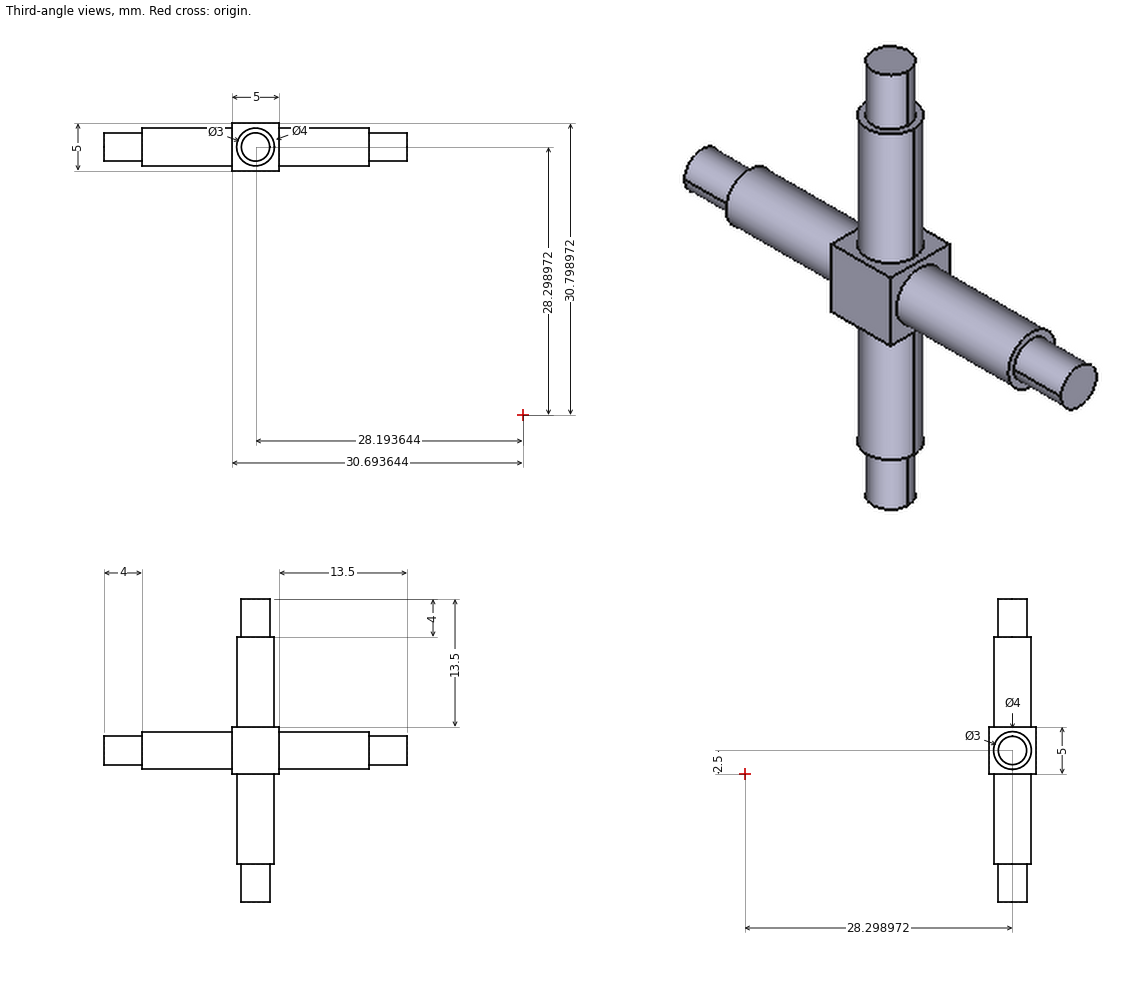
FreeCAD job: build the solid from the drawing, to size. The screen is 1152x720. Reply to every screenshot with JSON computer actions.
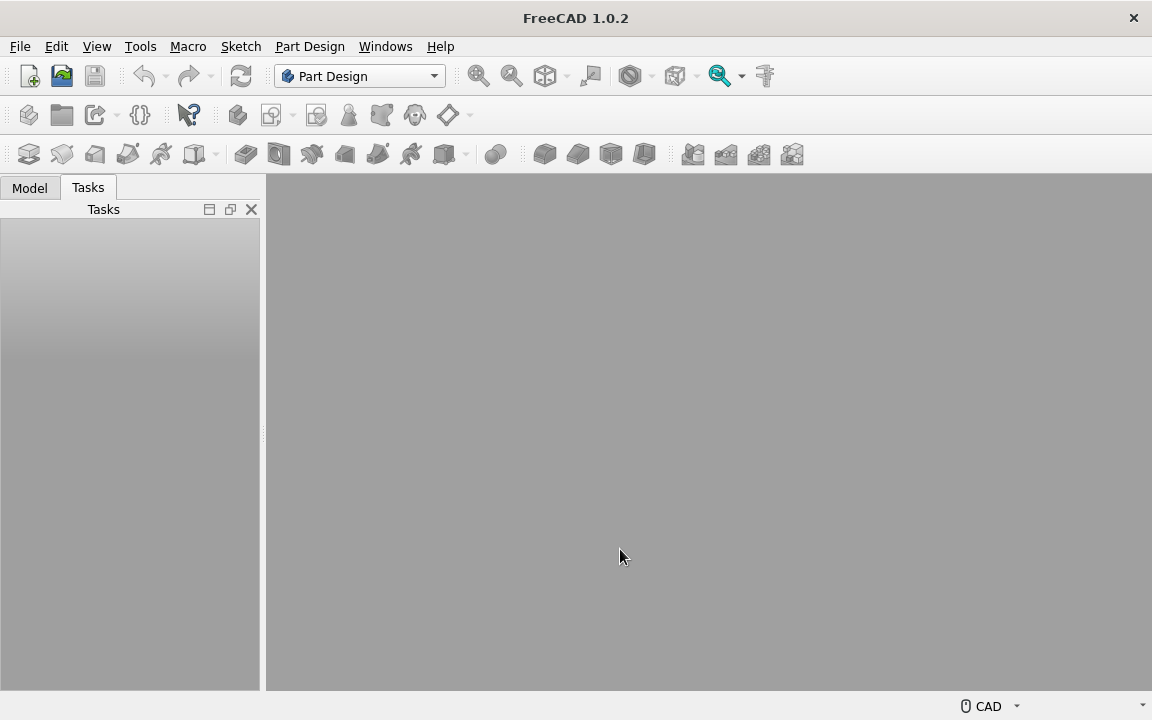
{"action": "left_click", "coordinate": [29, 76]}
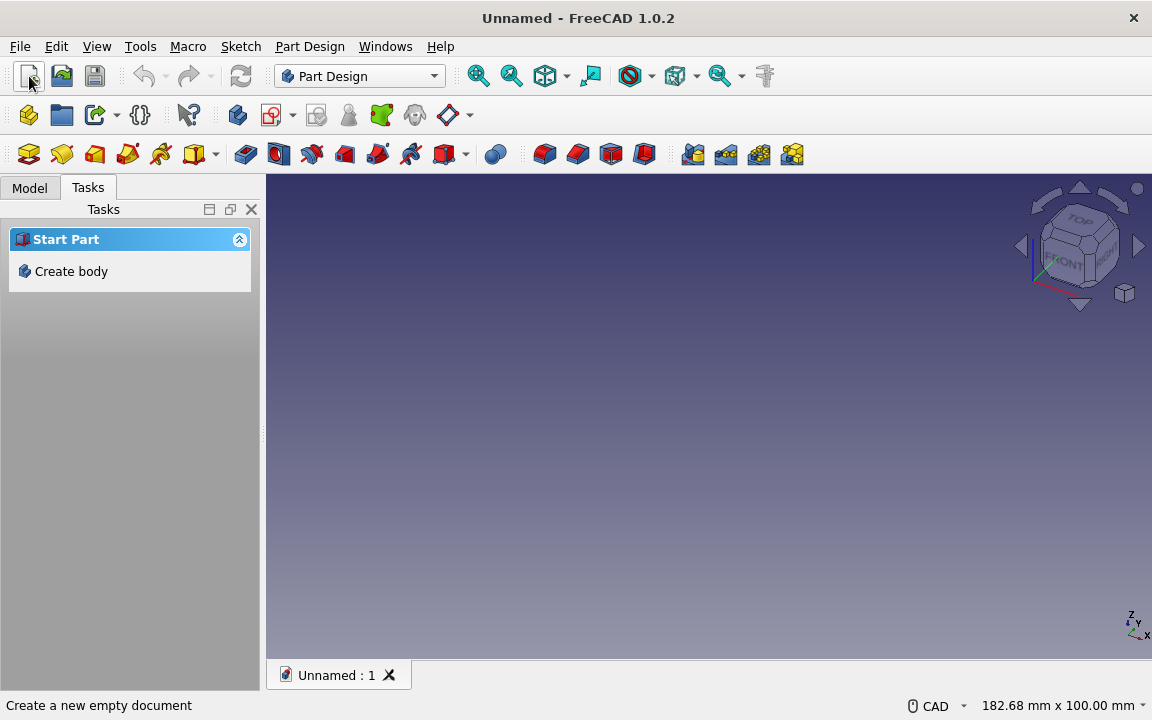
{"action": "left_click", "coordinate": [270, 116]}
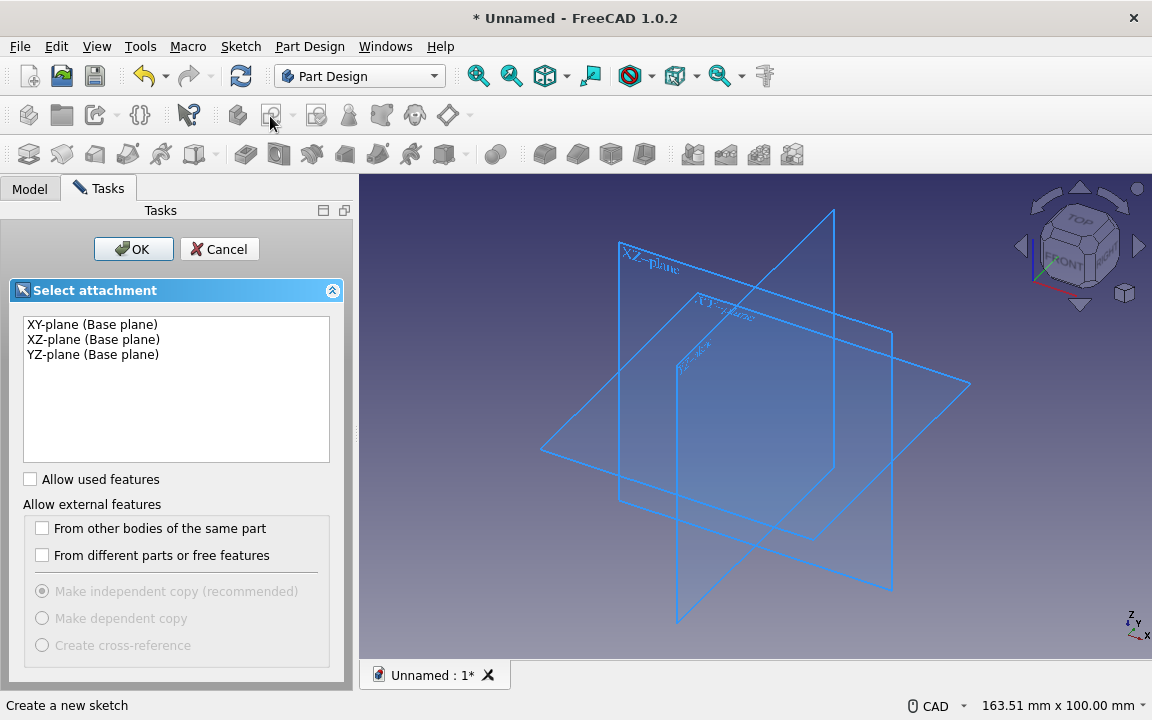
{"action": "left_click", "coordinate": [84, 324]}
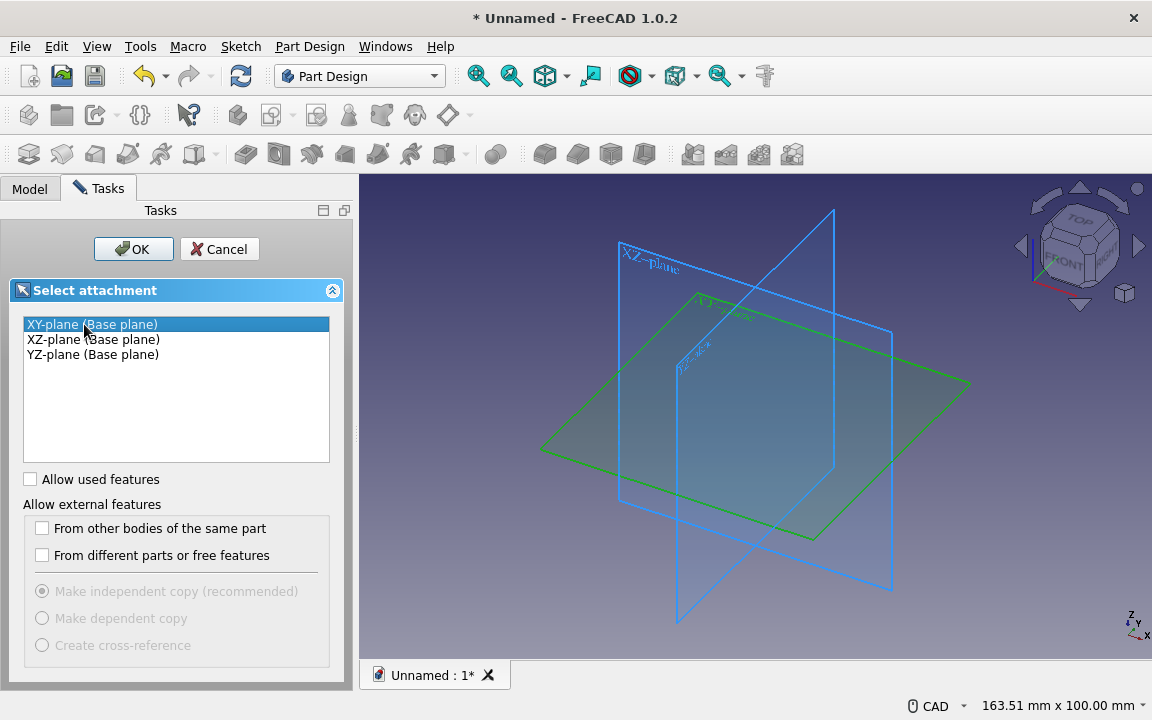
{"action": "left_click", "coordinate": [134, 249]}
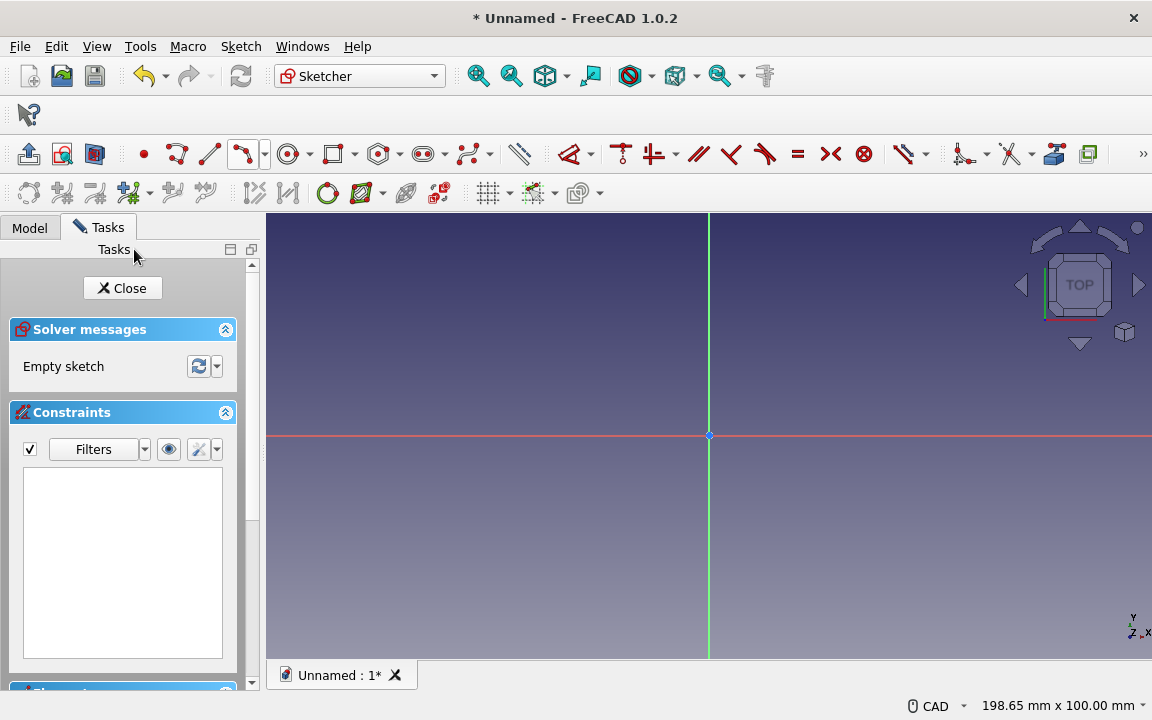
{"action": "scroll", "coordinate": [579, 300], "scroll_direction": "up", "scroll_amount": 13}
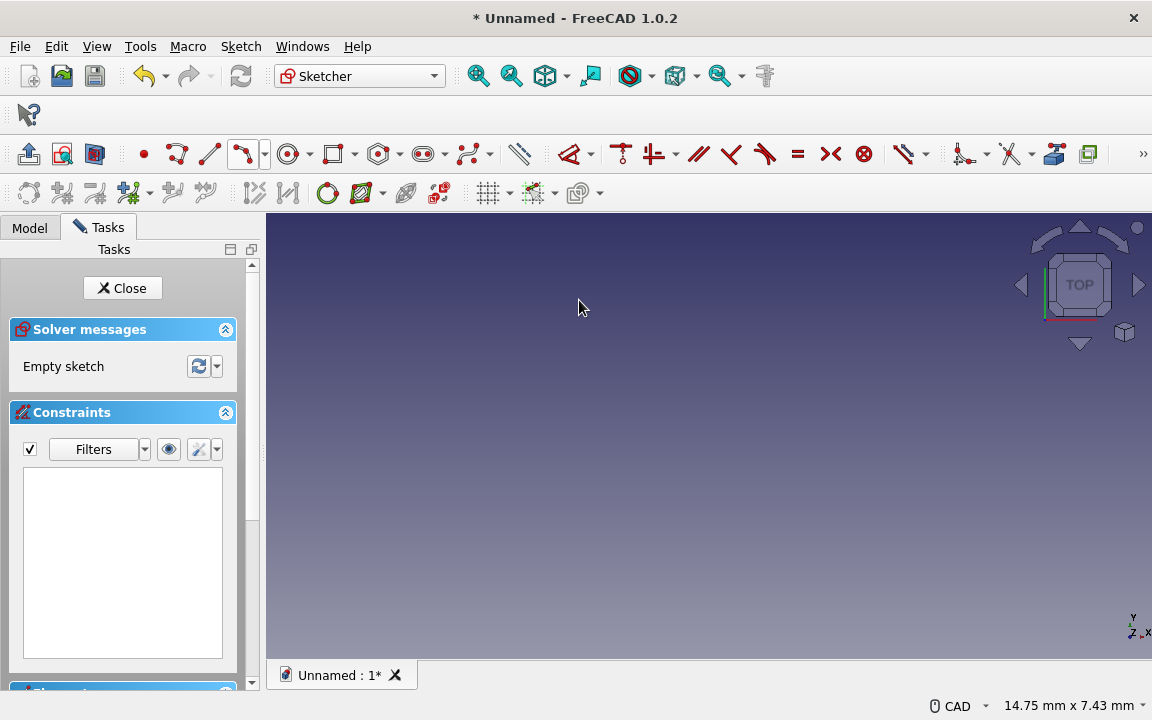
{"action": "left_click", "coordinate": [332, 154]}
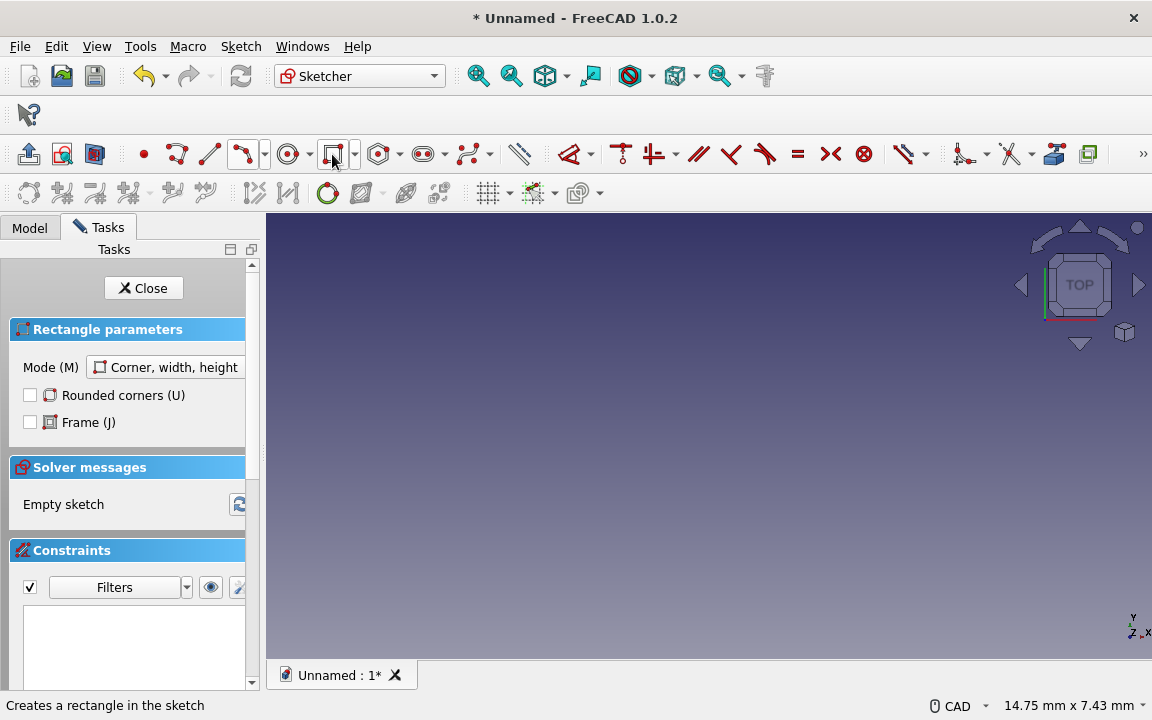
{"action": "left_click", "coordinate": [482, 279]}
{"action": "left_click", "coordinate": [782, 579]}
{"action": "key", "text": "Escape"}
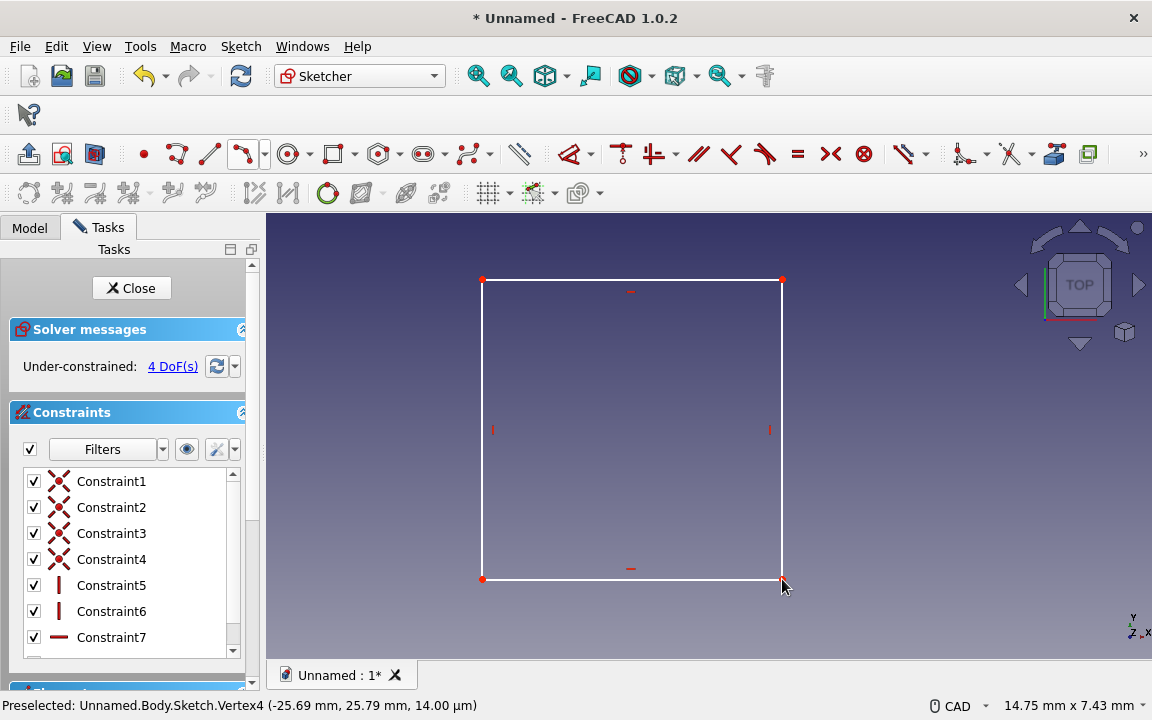
{"action": "left_click", "coordinate": [568, 154]}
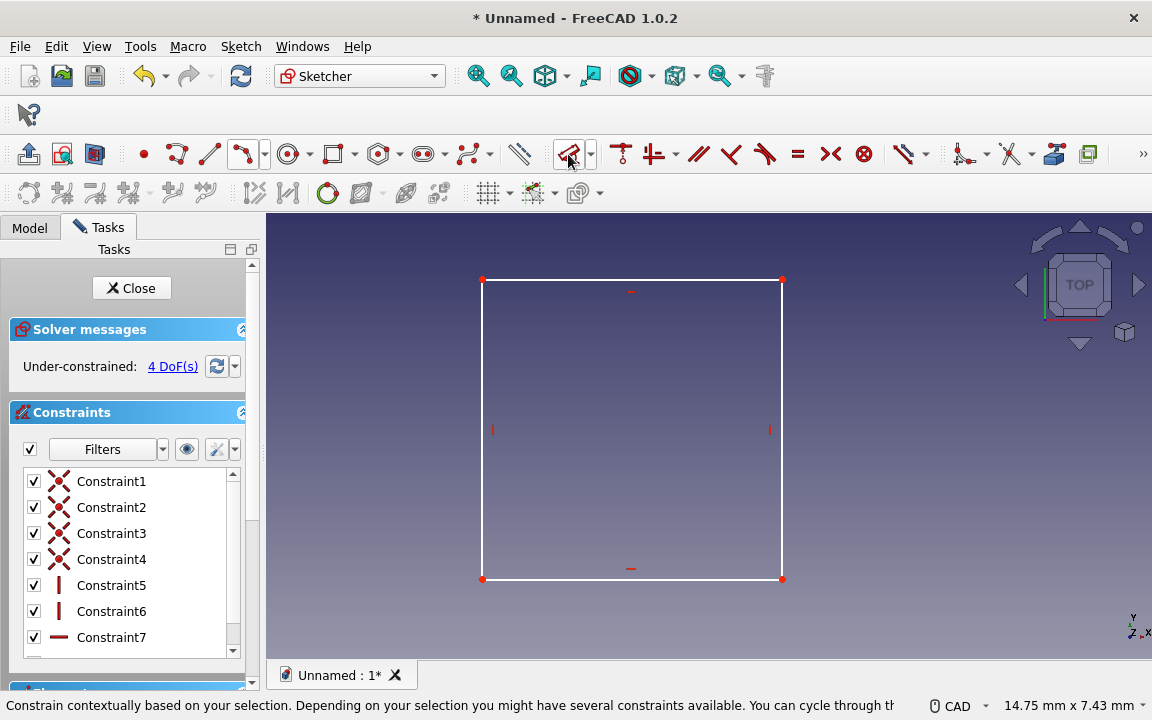
{"action": "left_click", "coordinate": [482, 370]}
{"action": "left_click", "coordinate": [448, 430]}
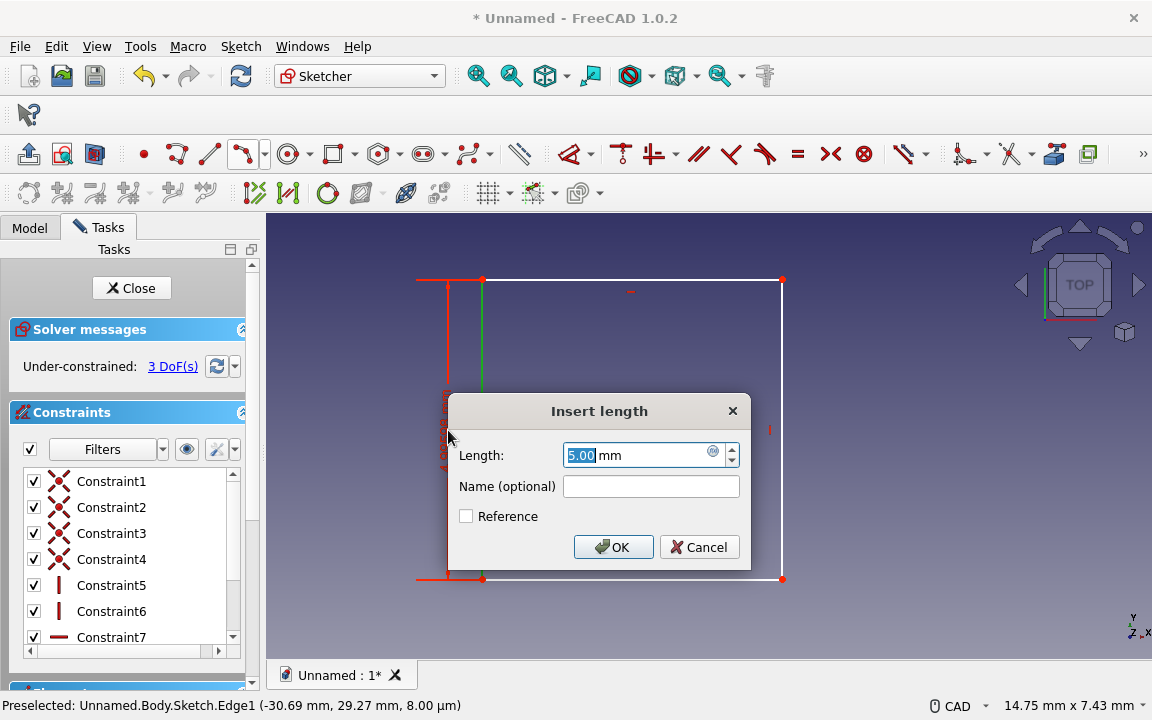
{"action": "type", "text": "5"}
{"action": "key", "text": "Return"}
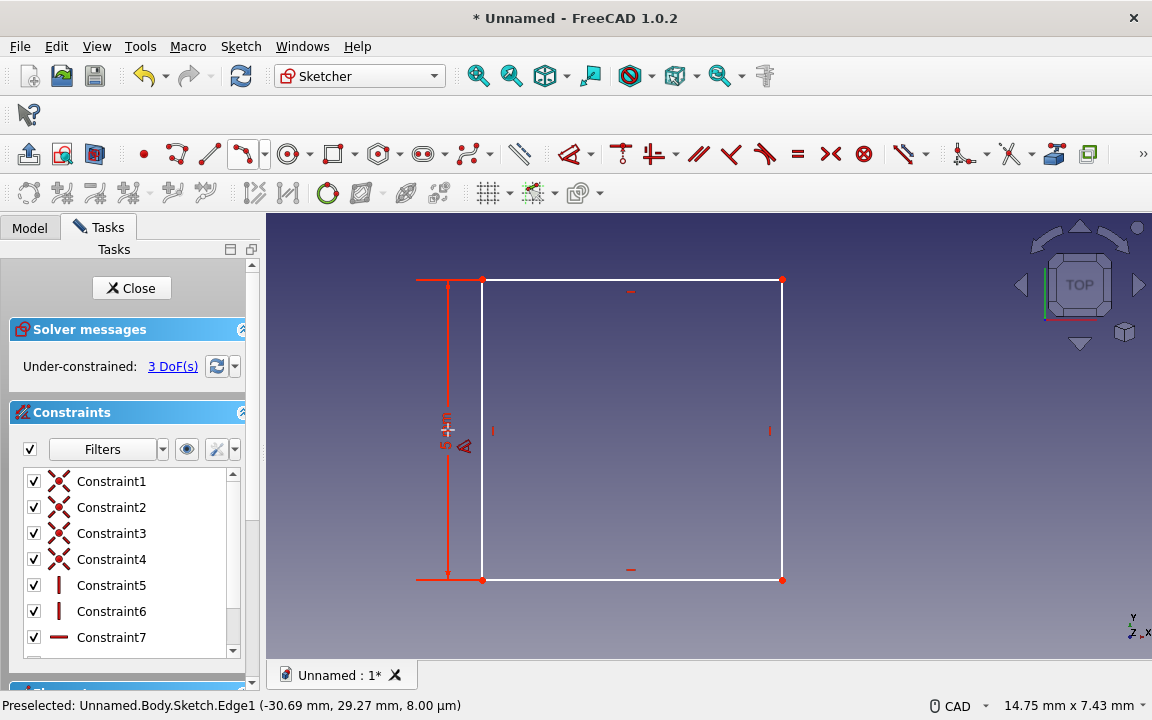
{"action": "left_click", "coordinate": [572, 580]}
{"action": "left_click", "coordinate": [632, 614]}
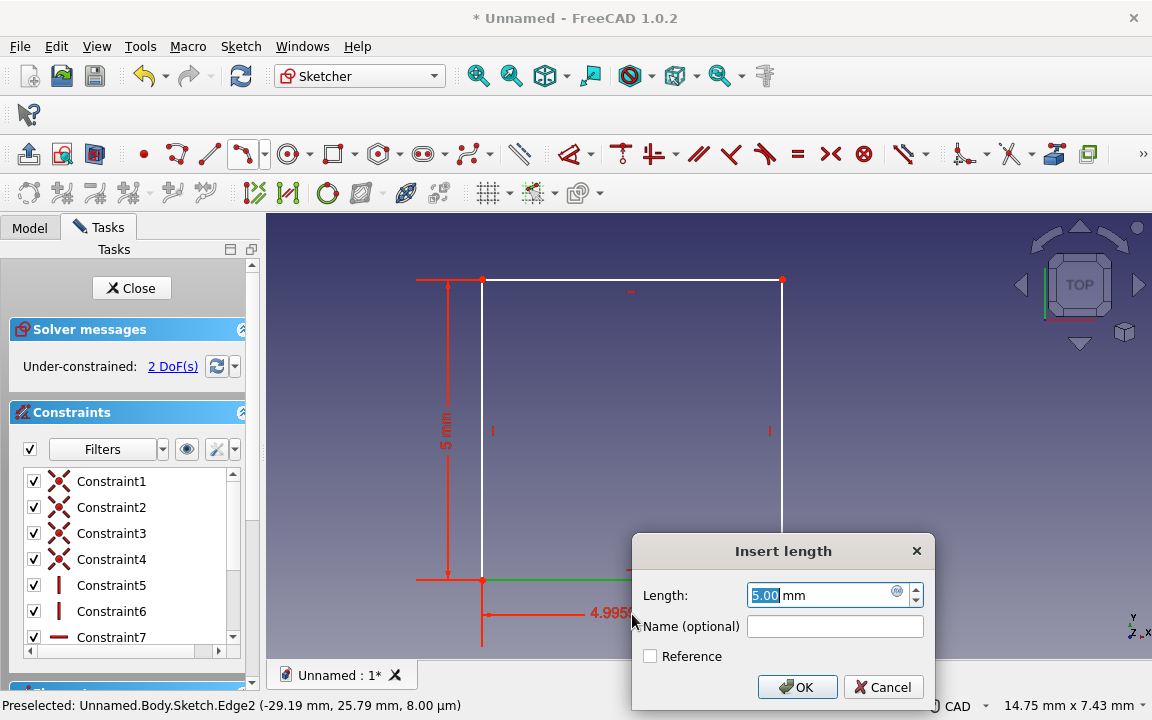
{"action": "type", "text": "5"}
{"action": "key", "text": "Return"}